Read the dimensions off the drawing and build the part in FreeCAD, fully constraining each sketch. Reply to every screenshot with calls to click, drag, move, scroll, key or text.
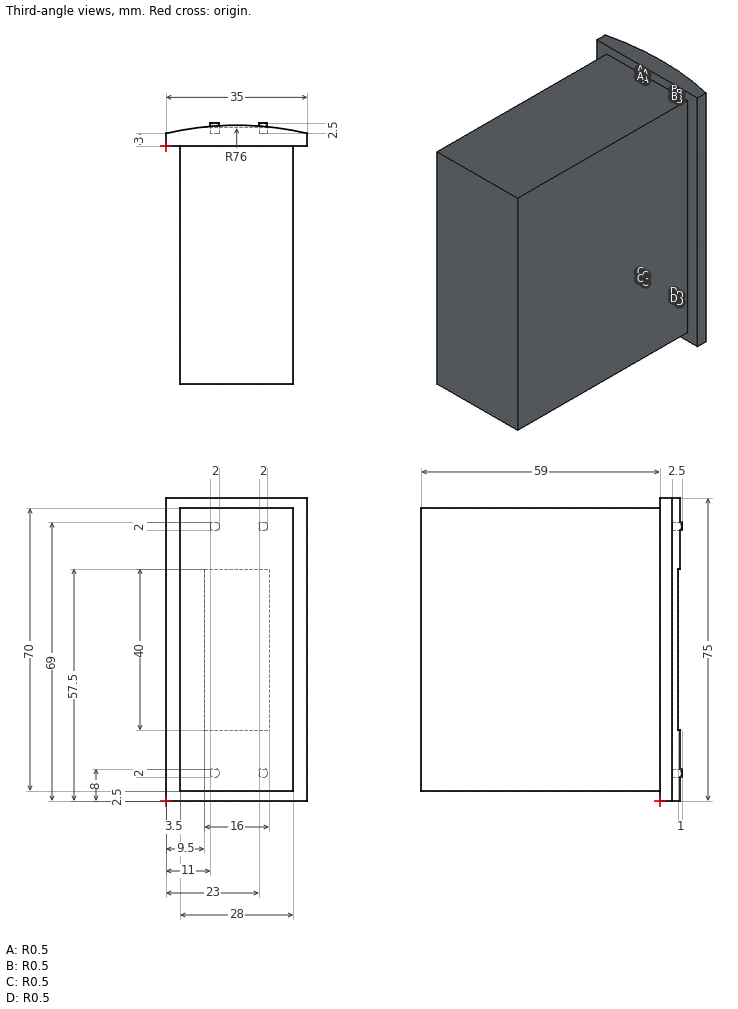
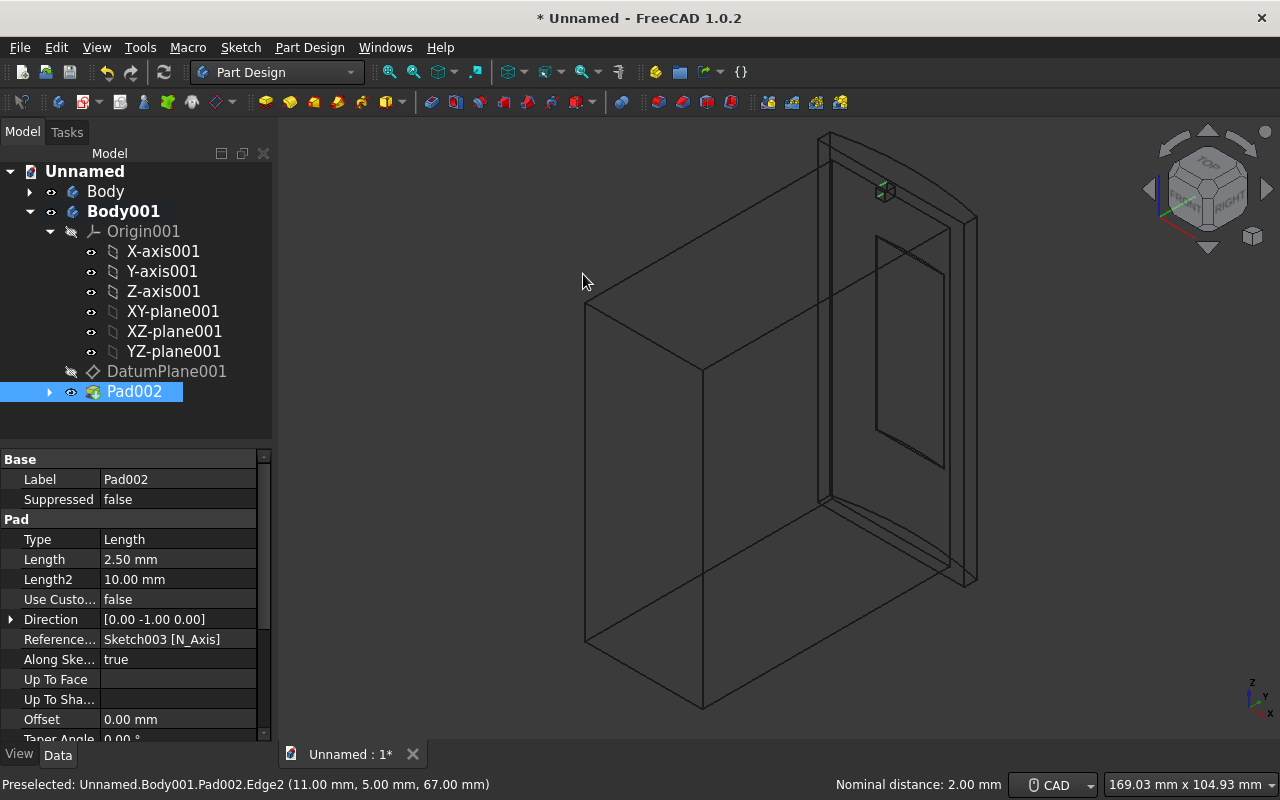
click(390, 72)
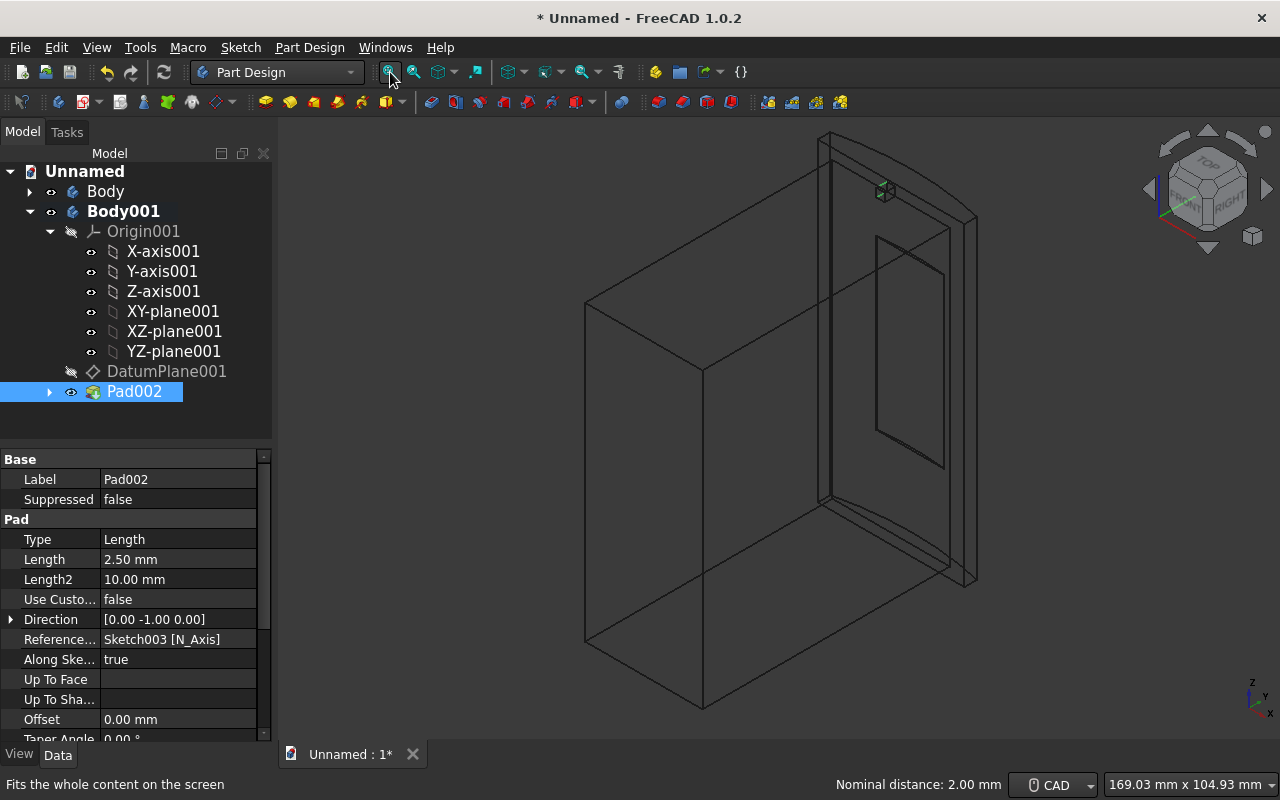
scroll(890, 189, up, 5)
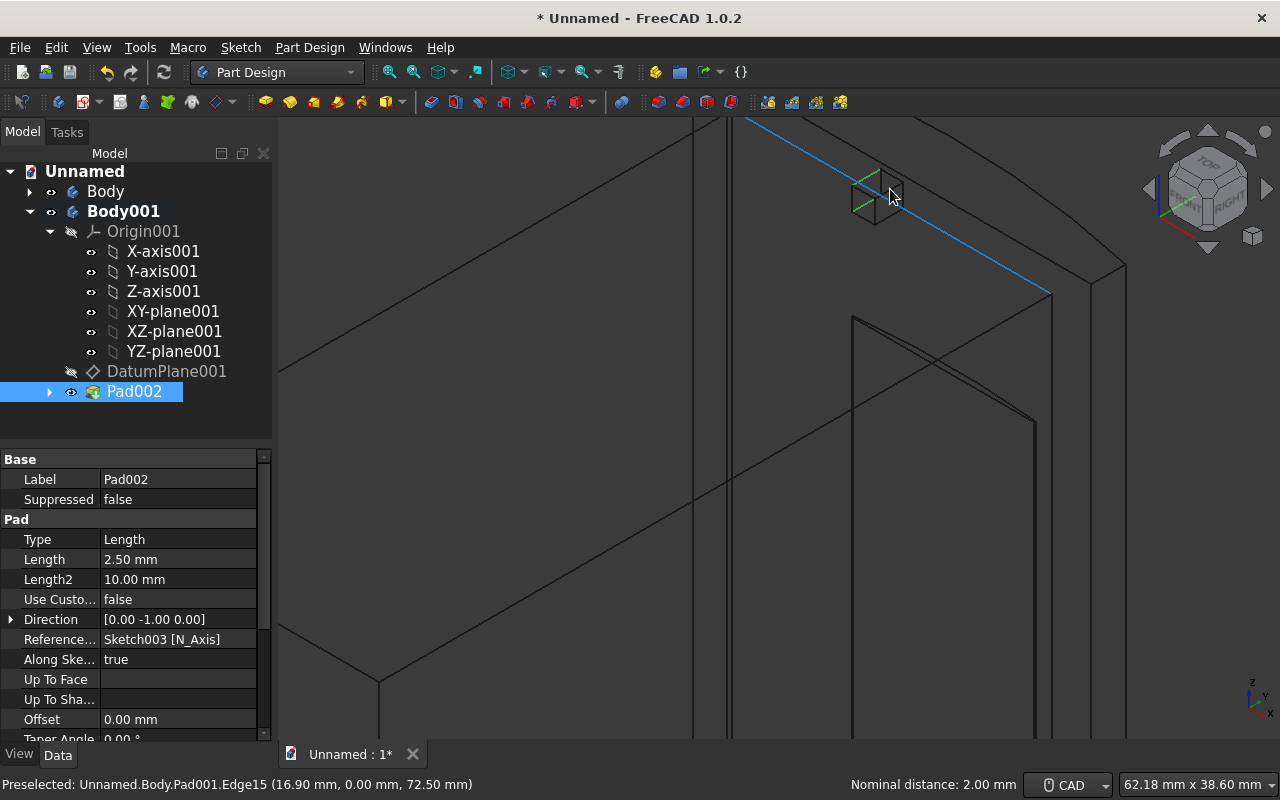
click(889, 190, ctrl)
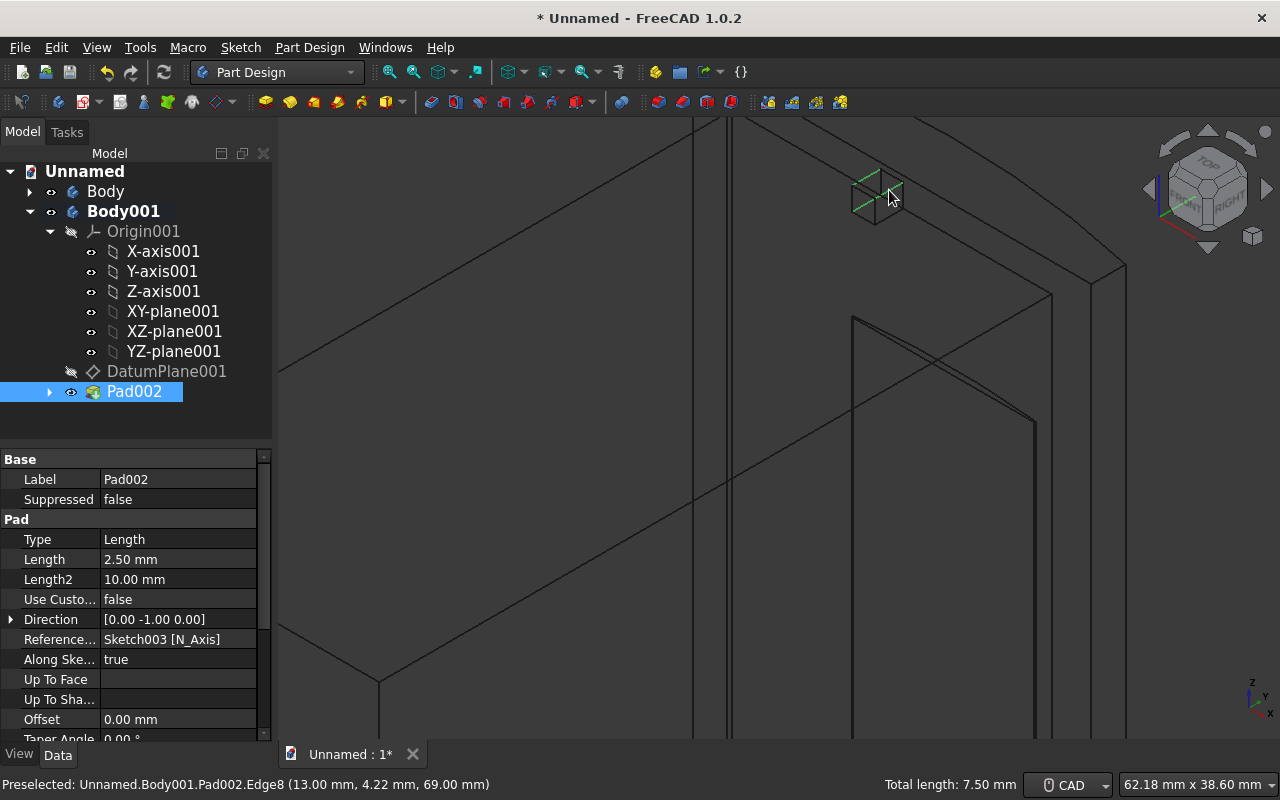
click(889, 216, ctrl)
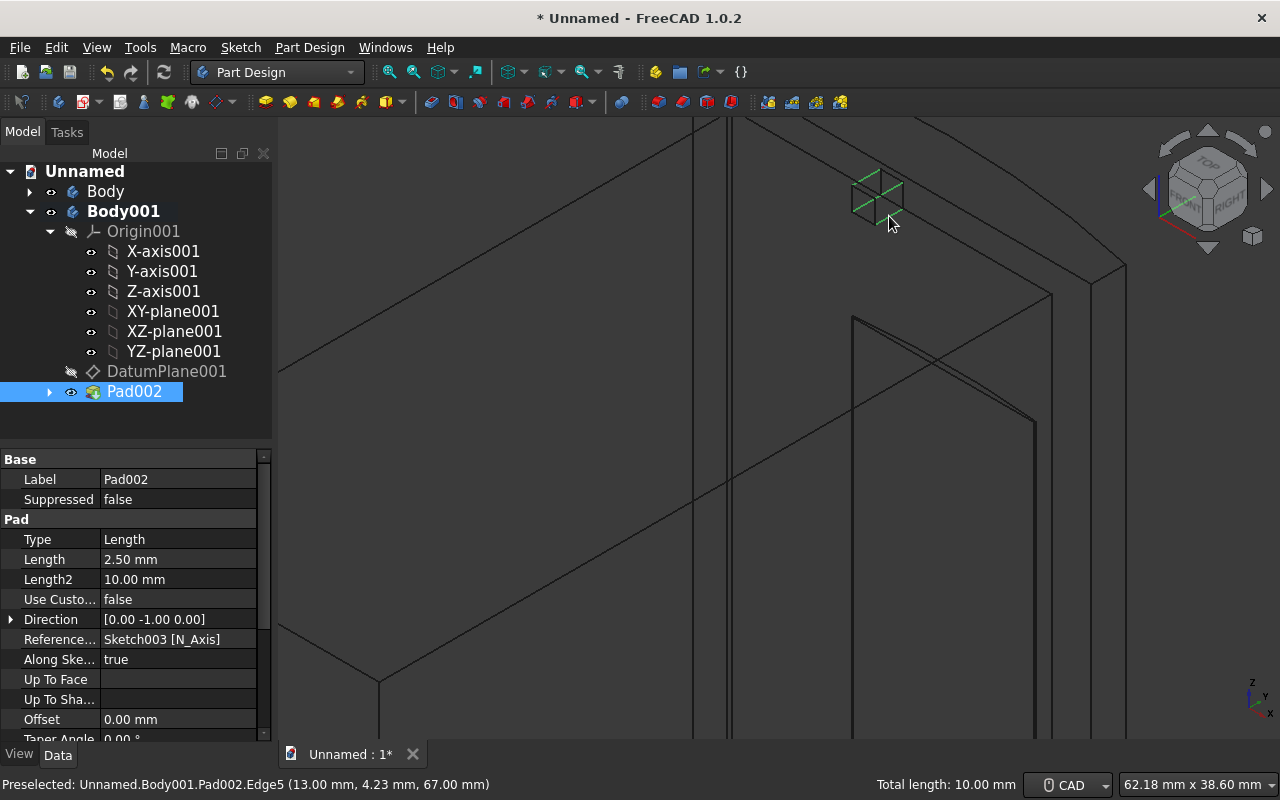
key(v)
key(1)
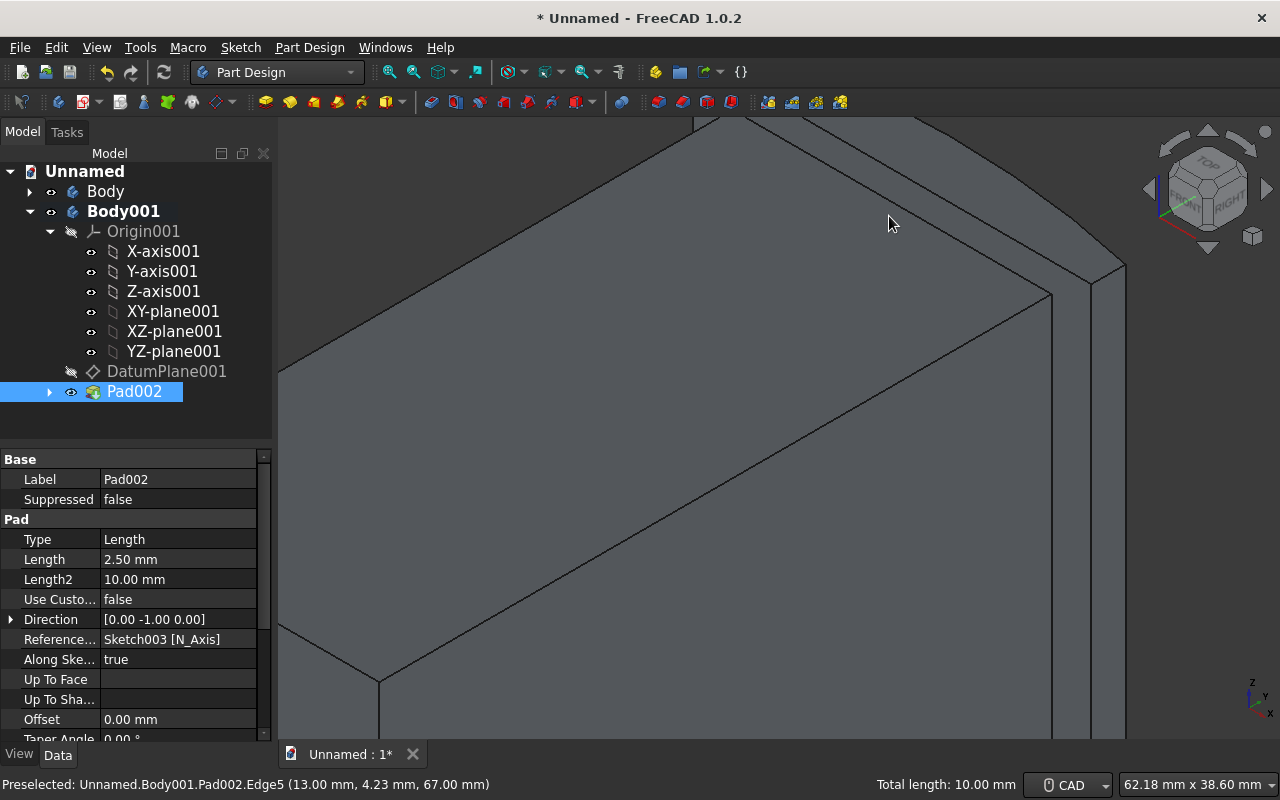
click(660, 102)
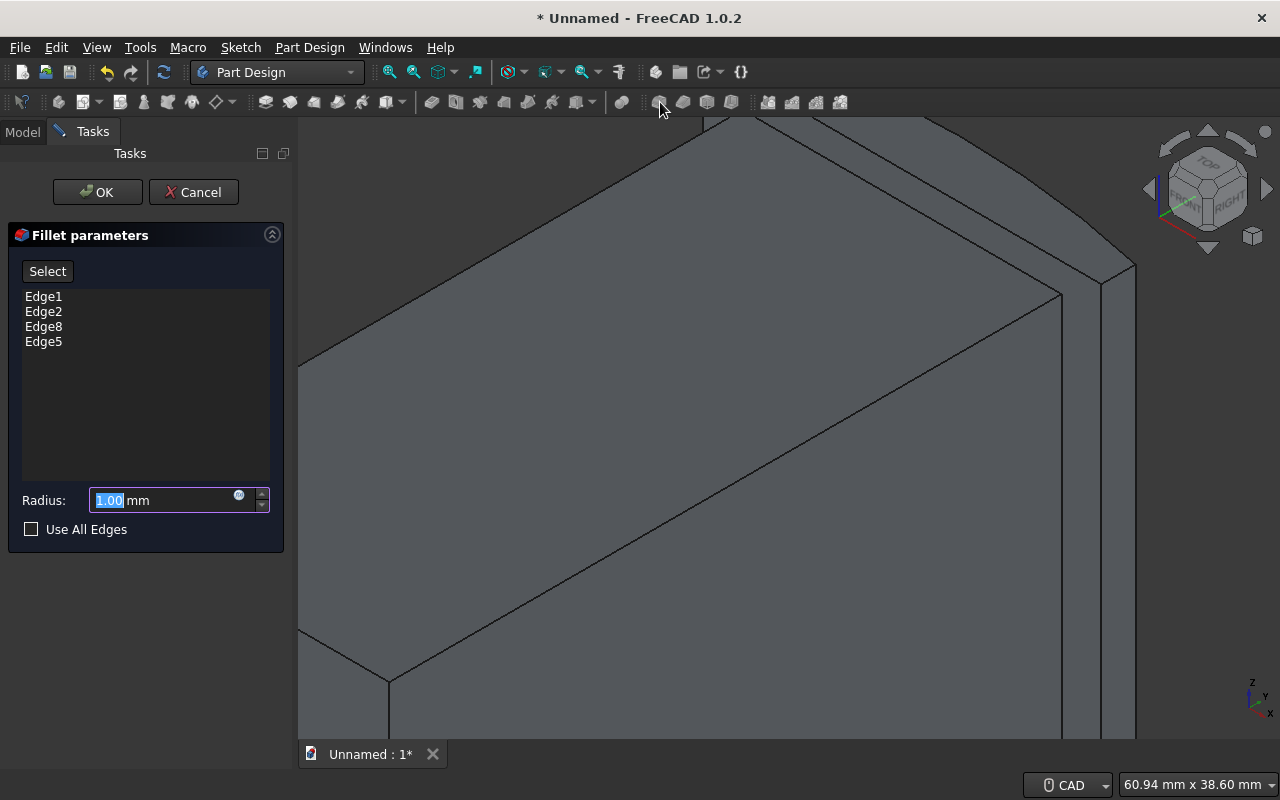
text(0.5)
key(Tab)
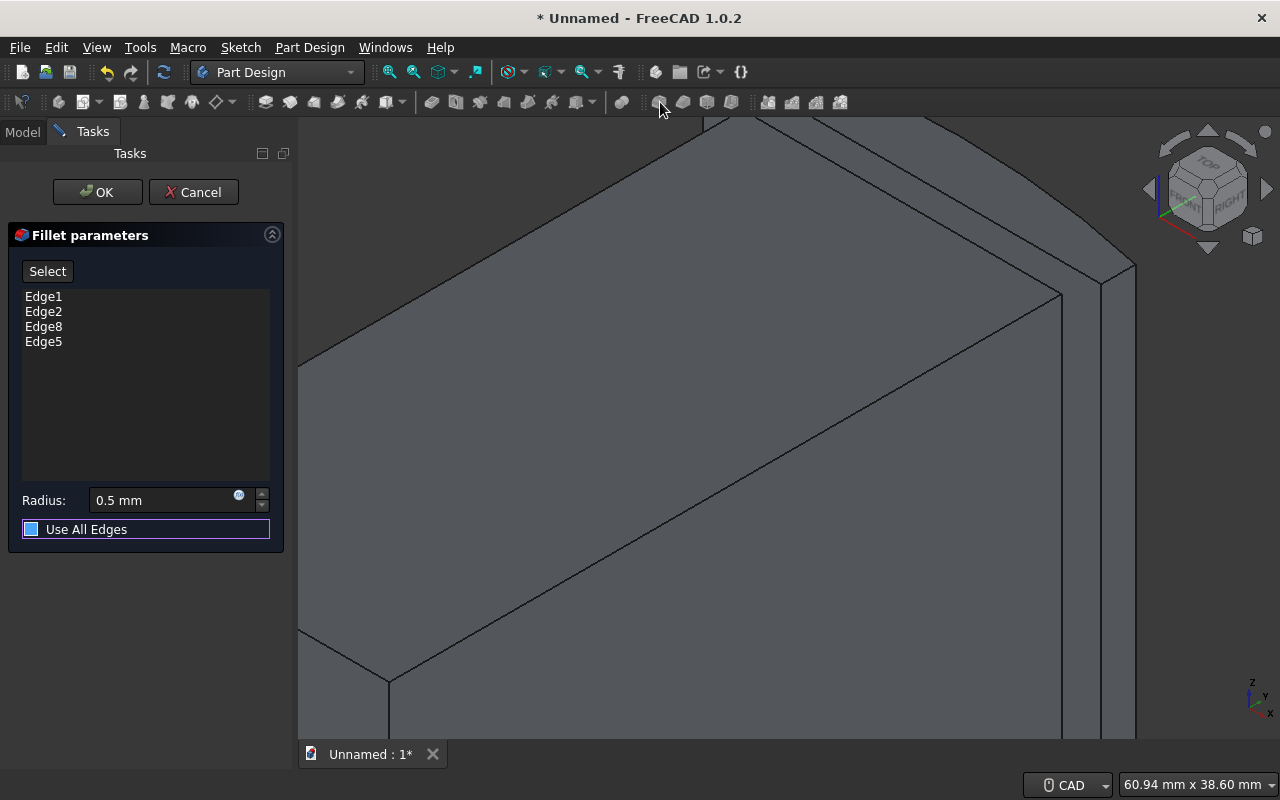
click(98, 192)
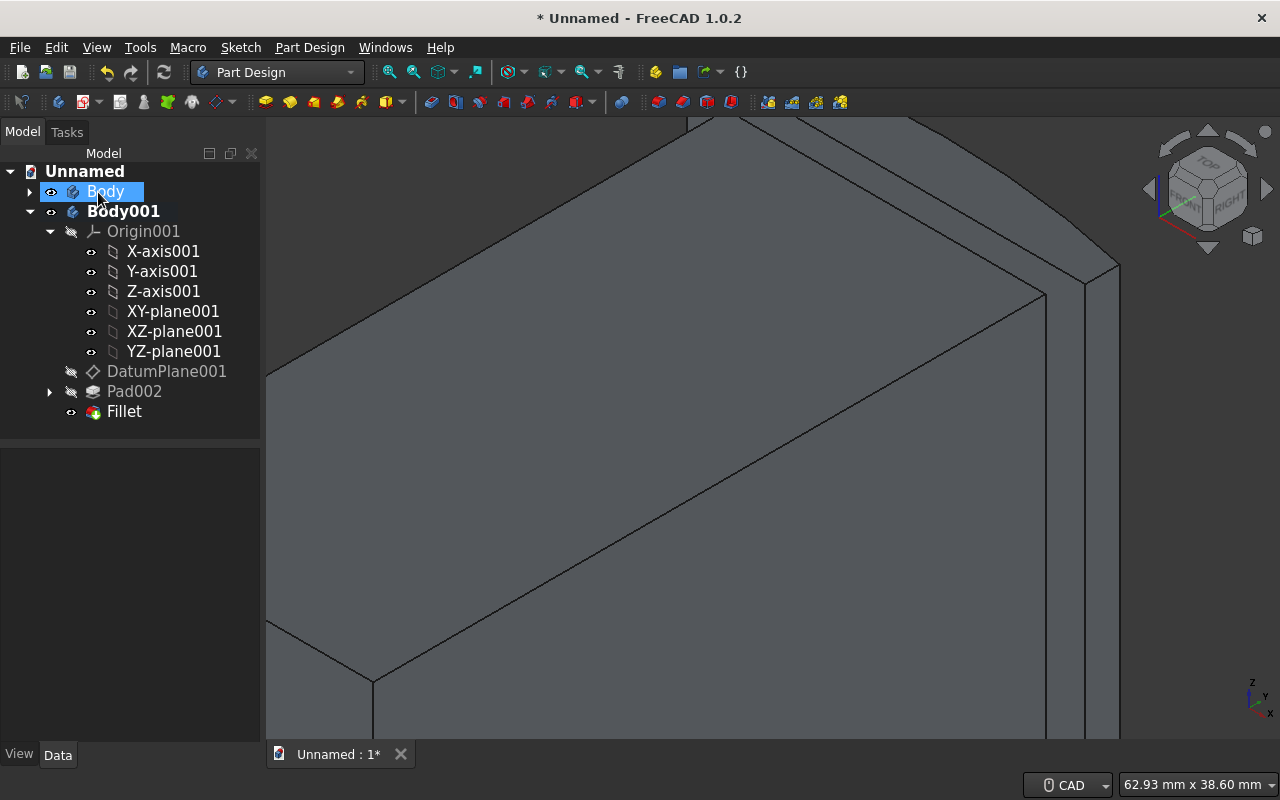
click(390, 72)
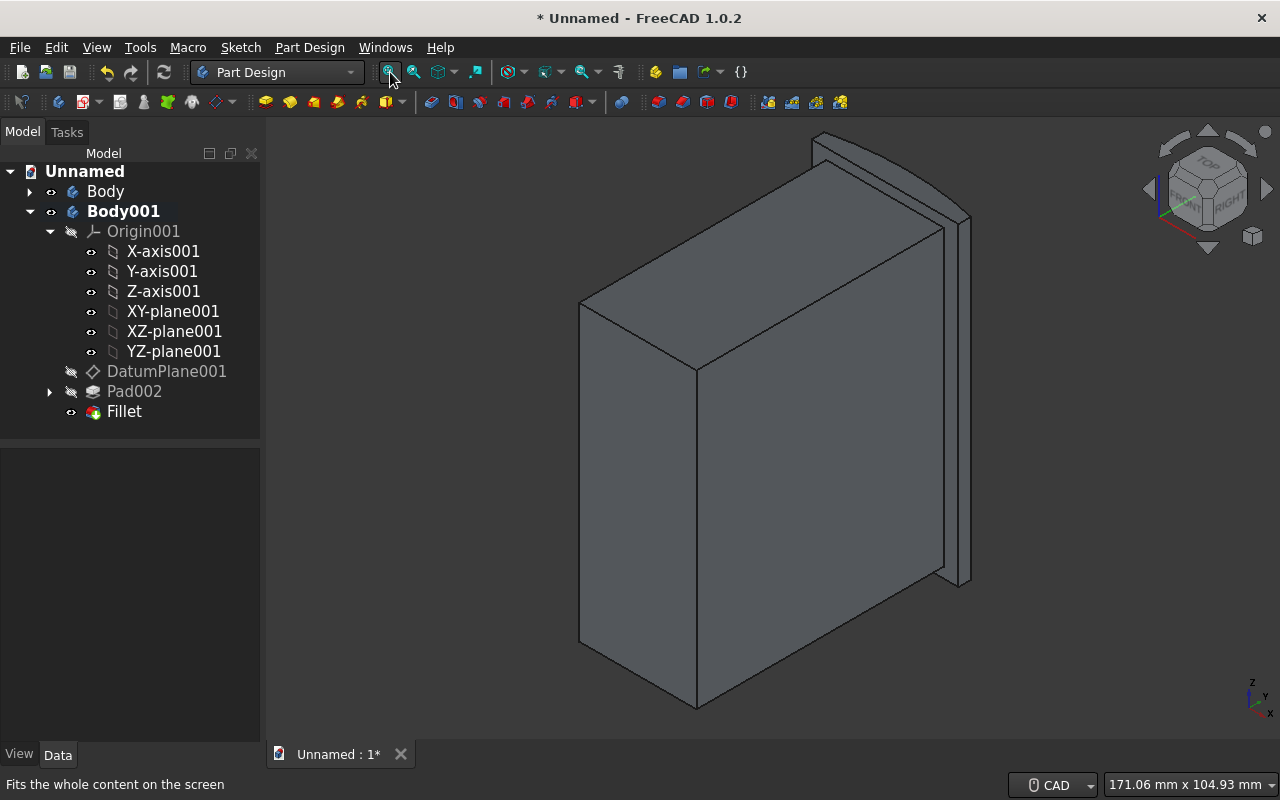
click(60, 102)